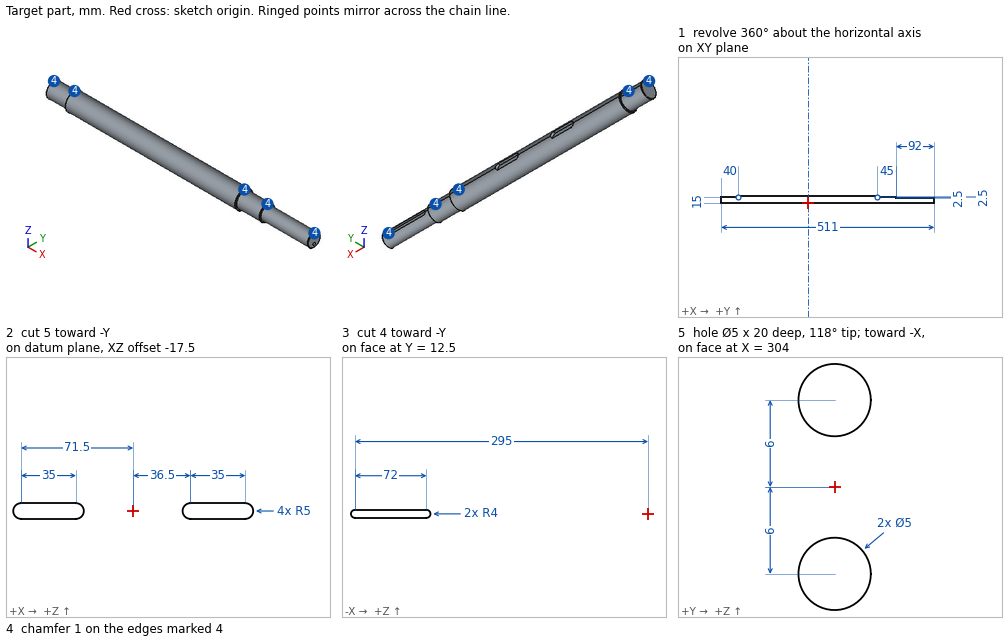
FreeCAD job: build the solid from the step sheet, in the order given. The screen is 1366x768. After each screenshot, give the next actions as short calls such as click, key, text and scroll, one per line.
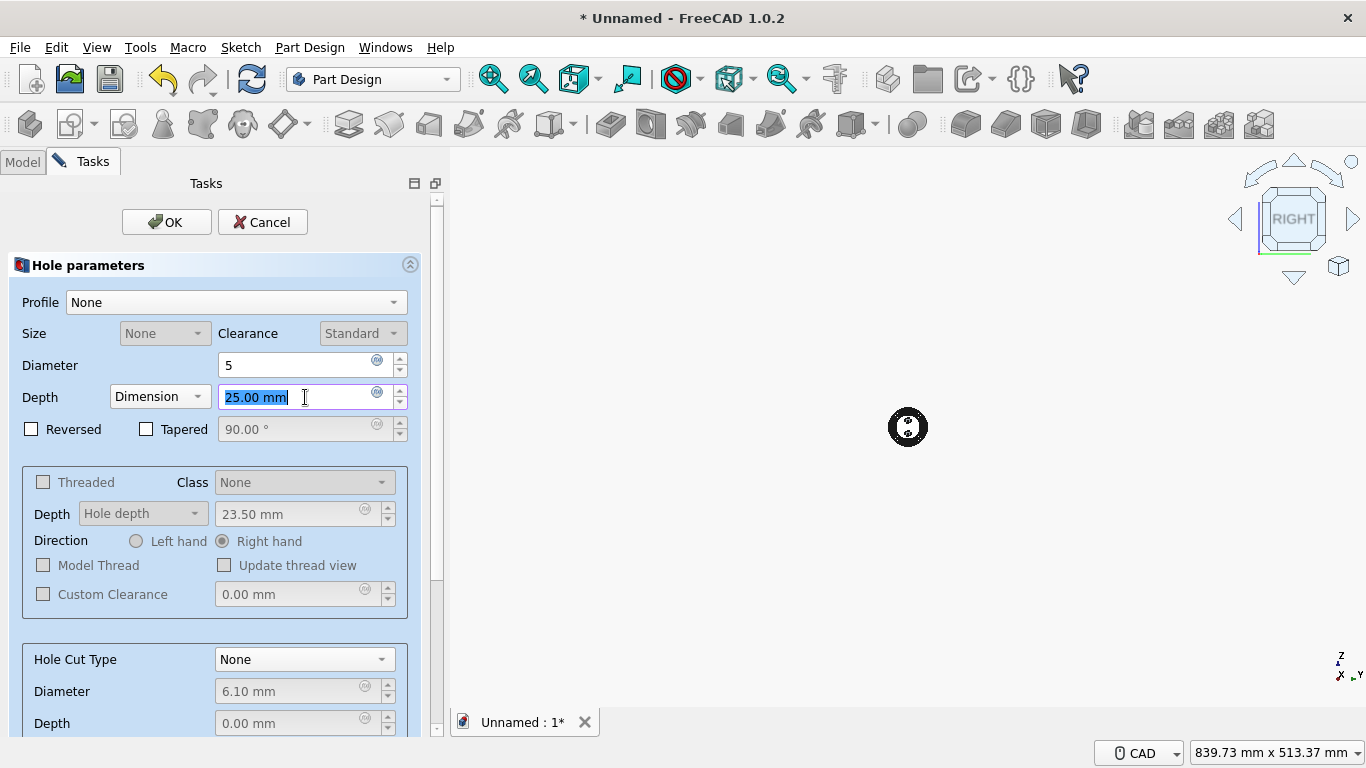
text(20)
key(Tab)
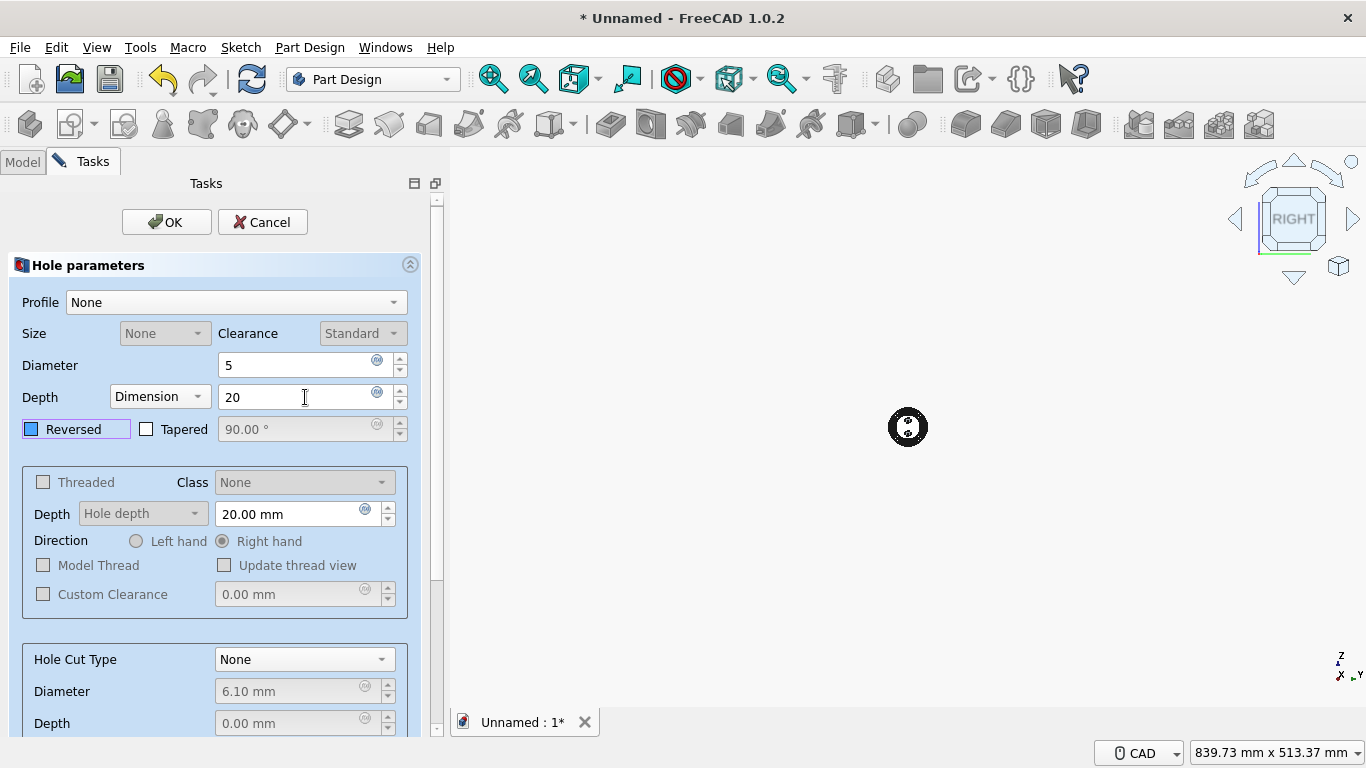
click(167, 222)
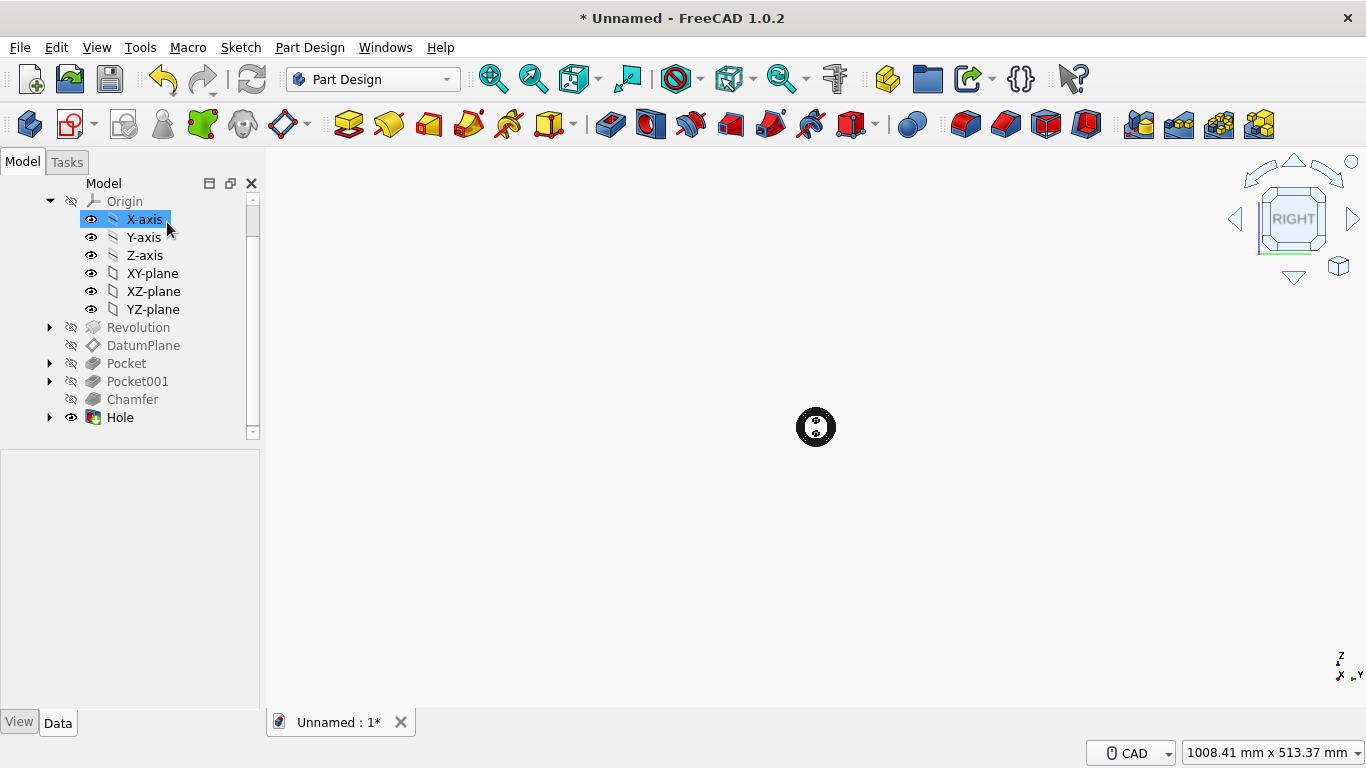
key(0)